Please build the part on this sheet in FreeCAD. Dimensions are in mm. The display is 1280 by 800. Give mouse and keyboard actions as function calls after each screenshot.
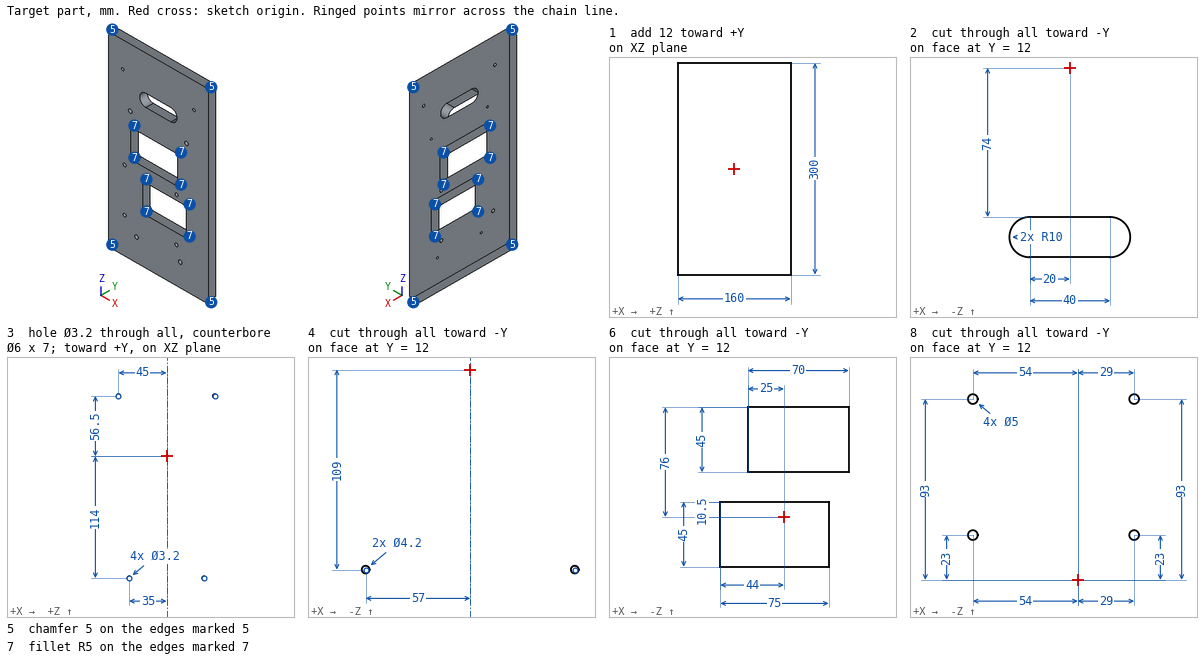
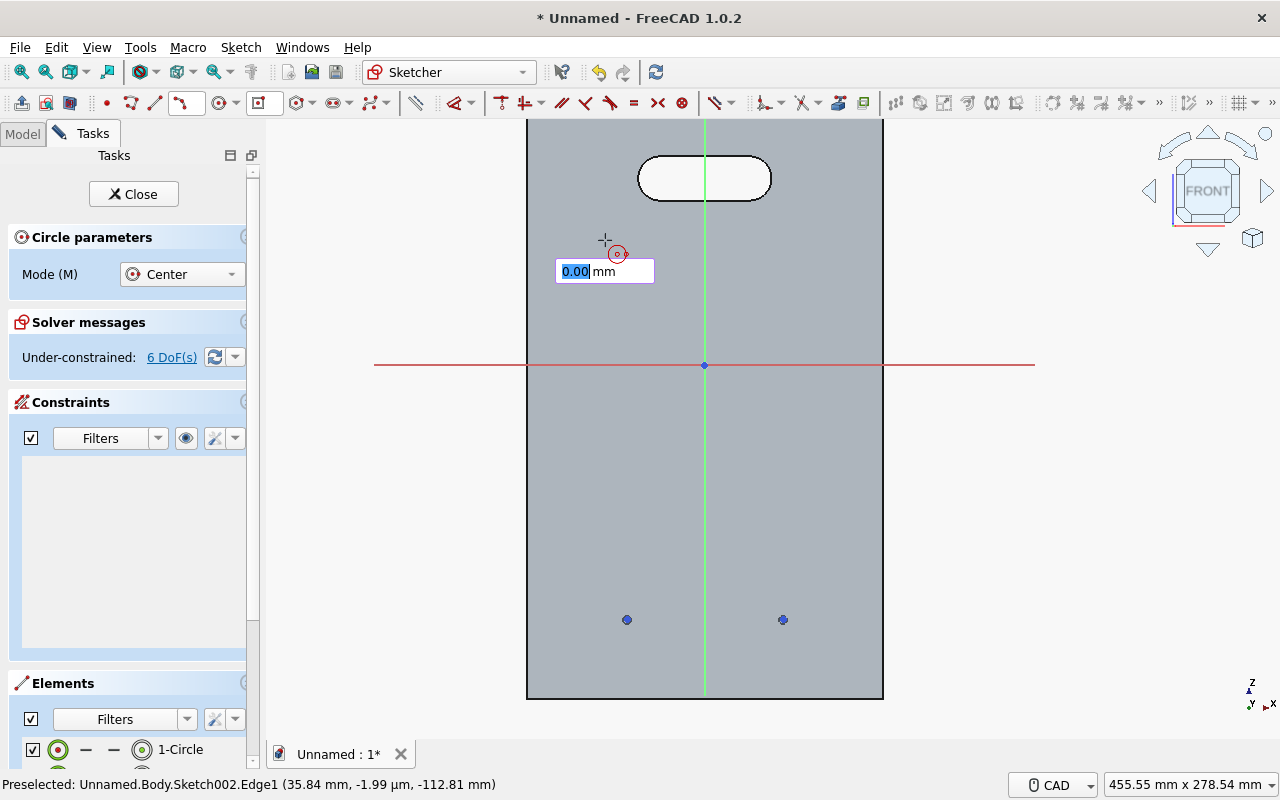
scroll(607, 237, up, 8)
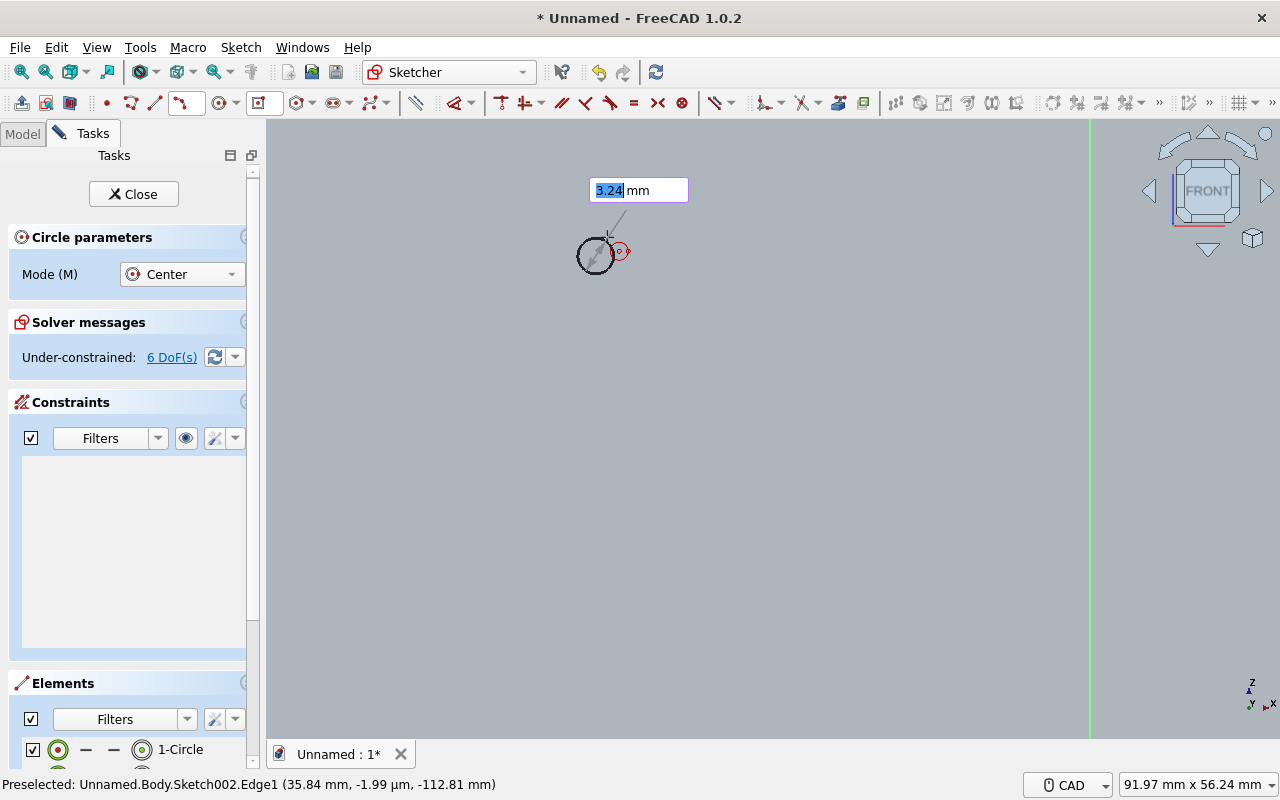
click(607, 237)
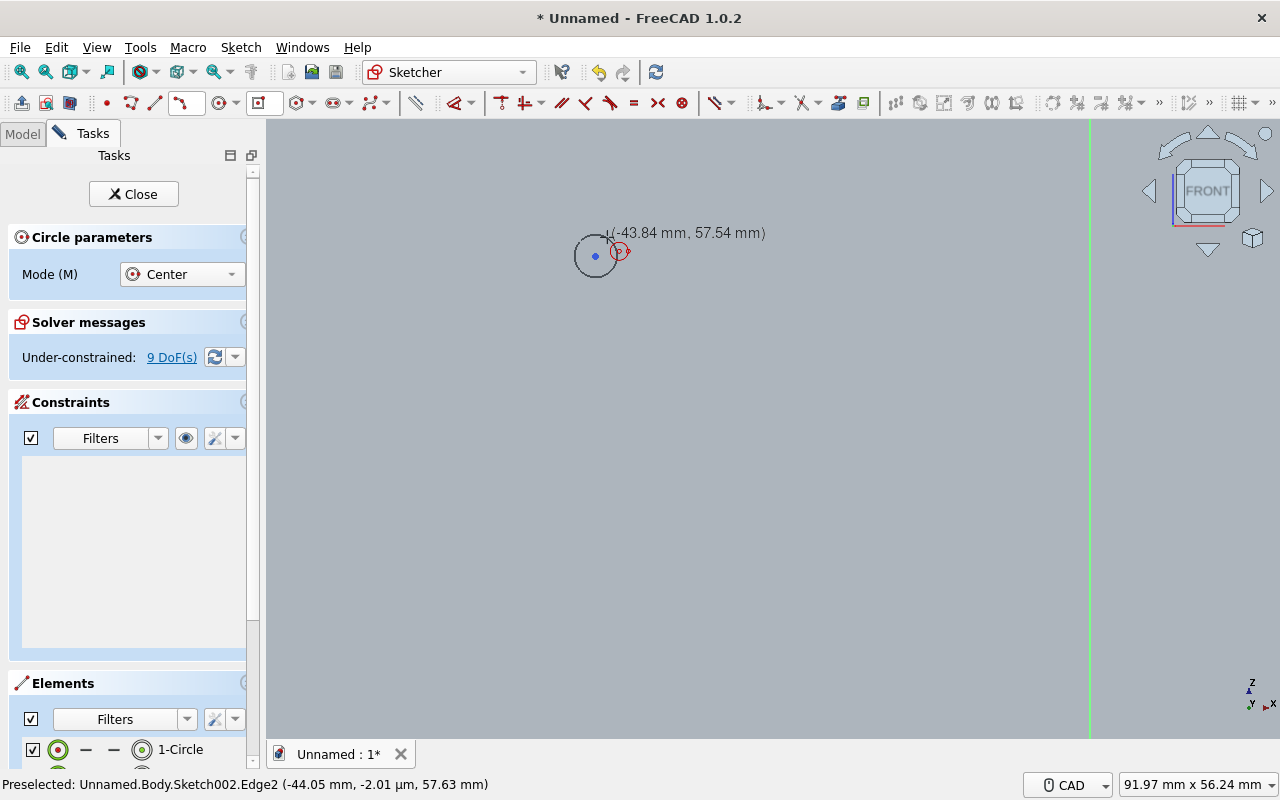
scroll(607, 237, down, 8)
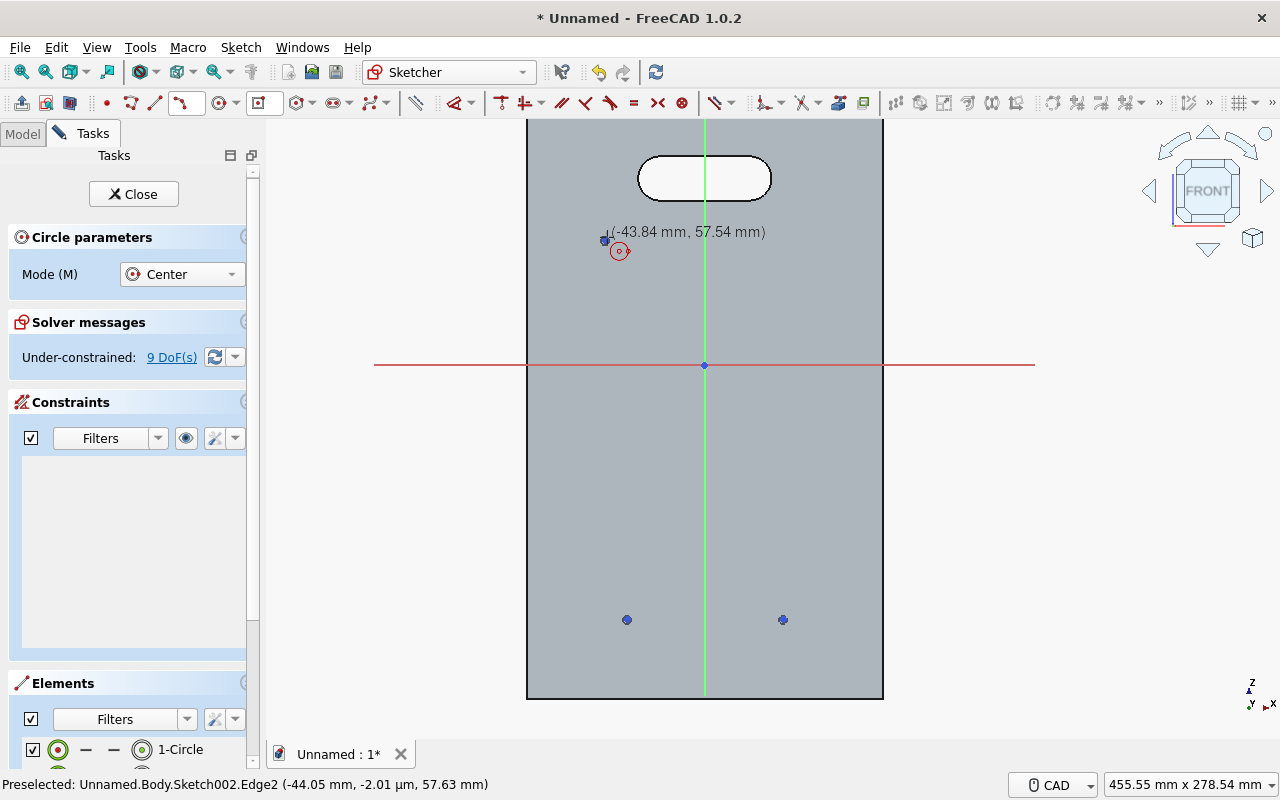
scroll(805, 240, up, 10)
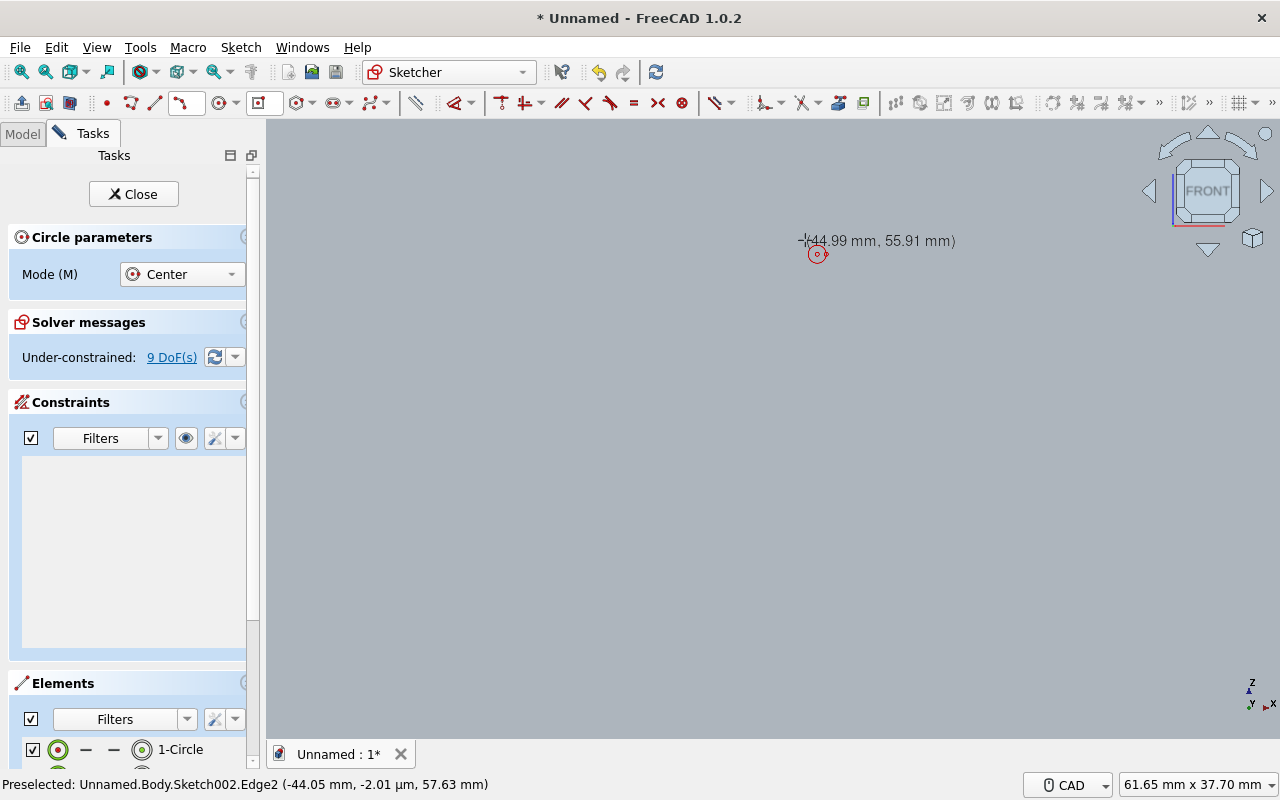
scroll(805, 240, down, 10)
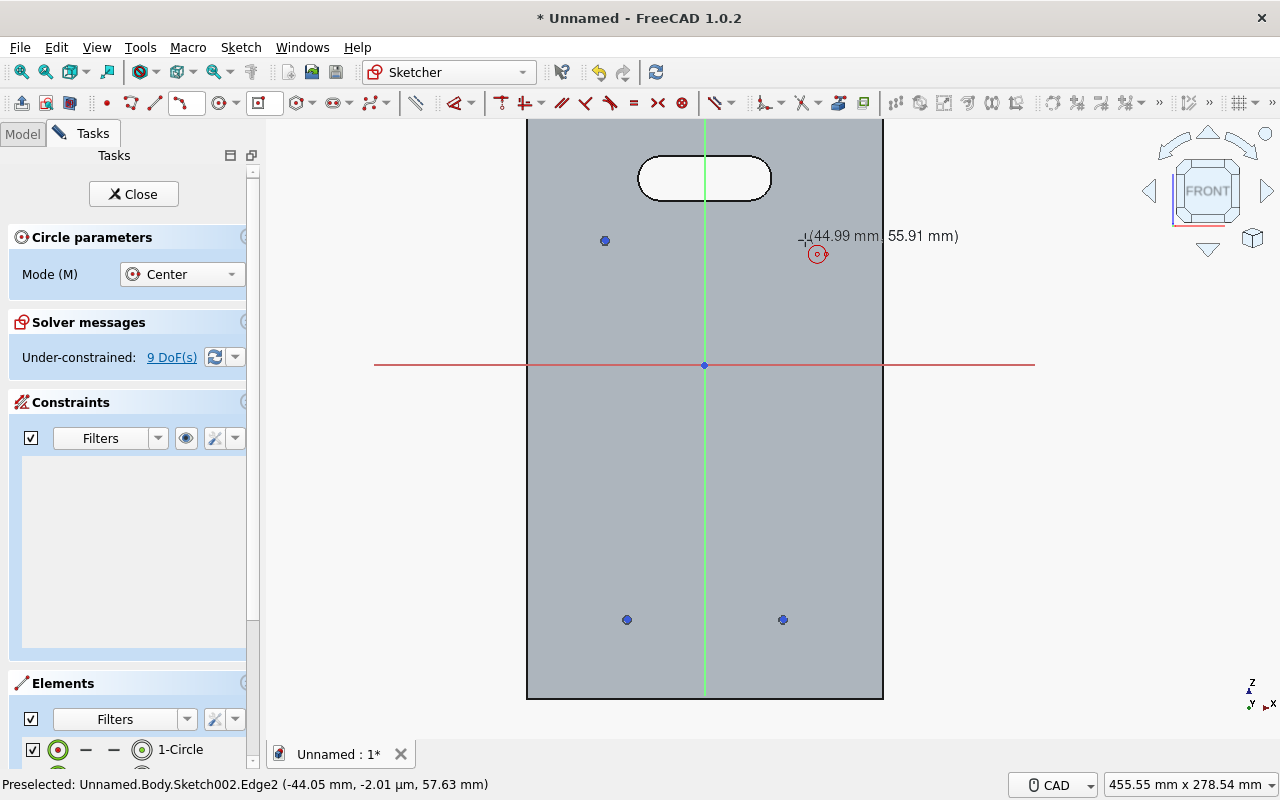
click(805, 240)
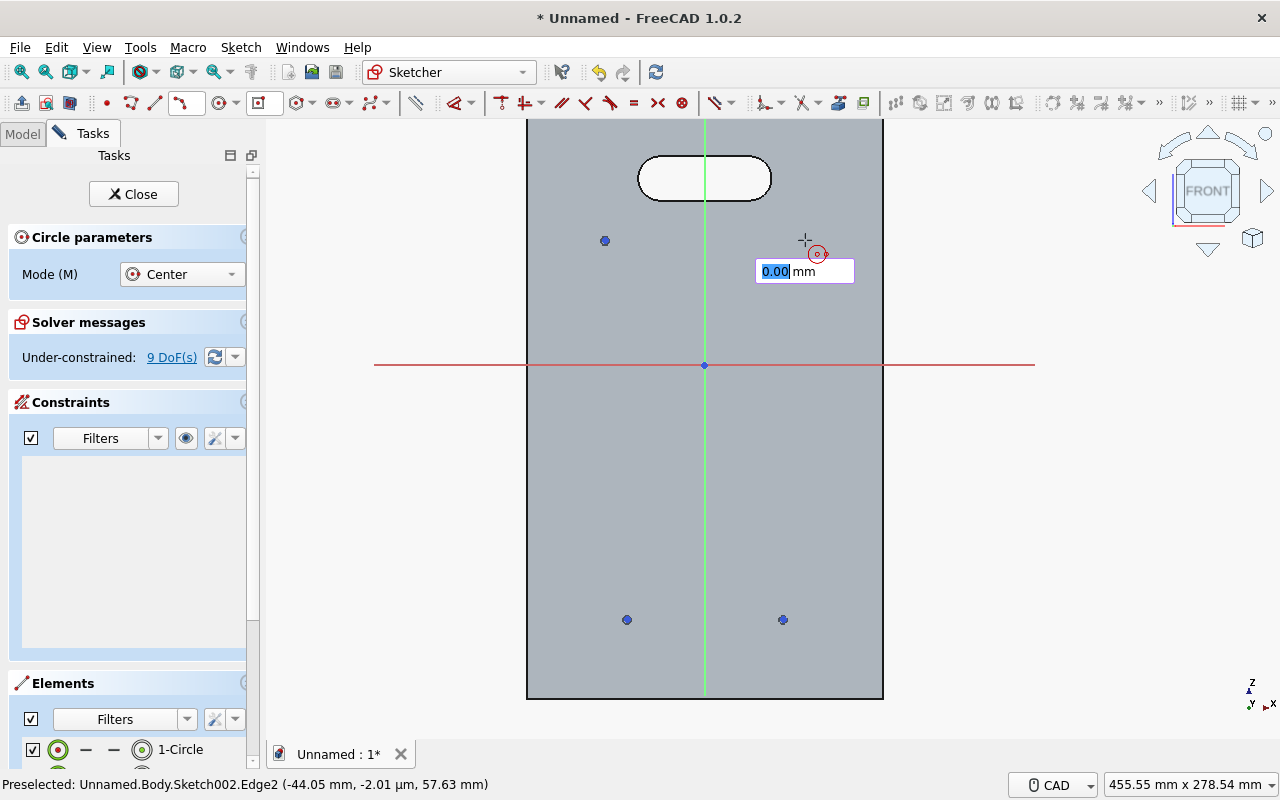
scroll(808, 237, up, 8)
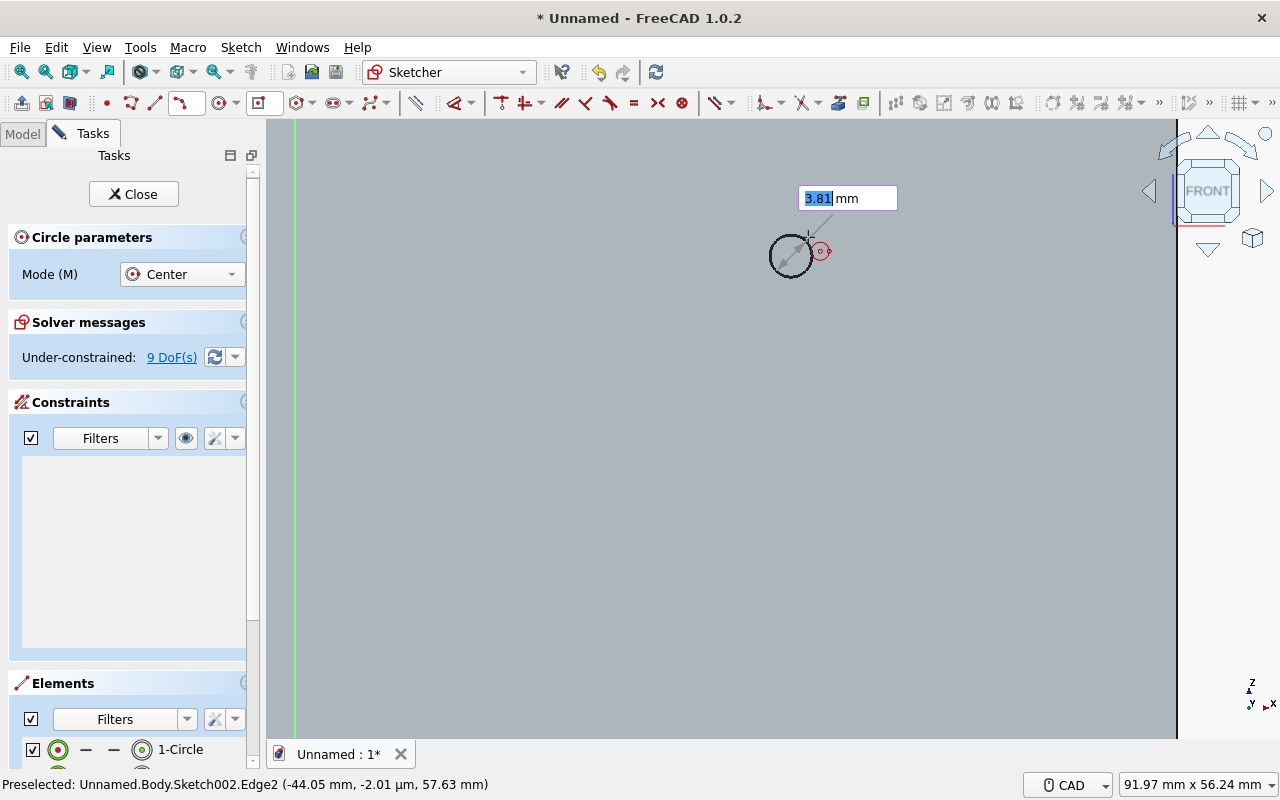
click(804, 237)
key(Escape)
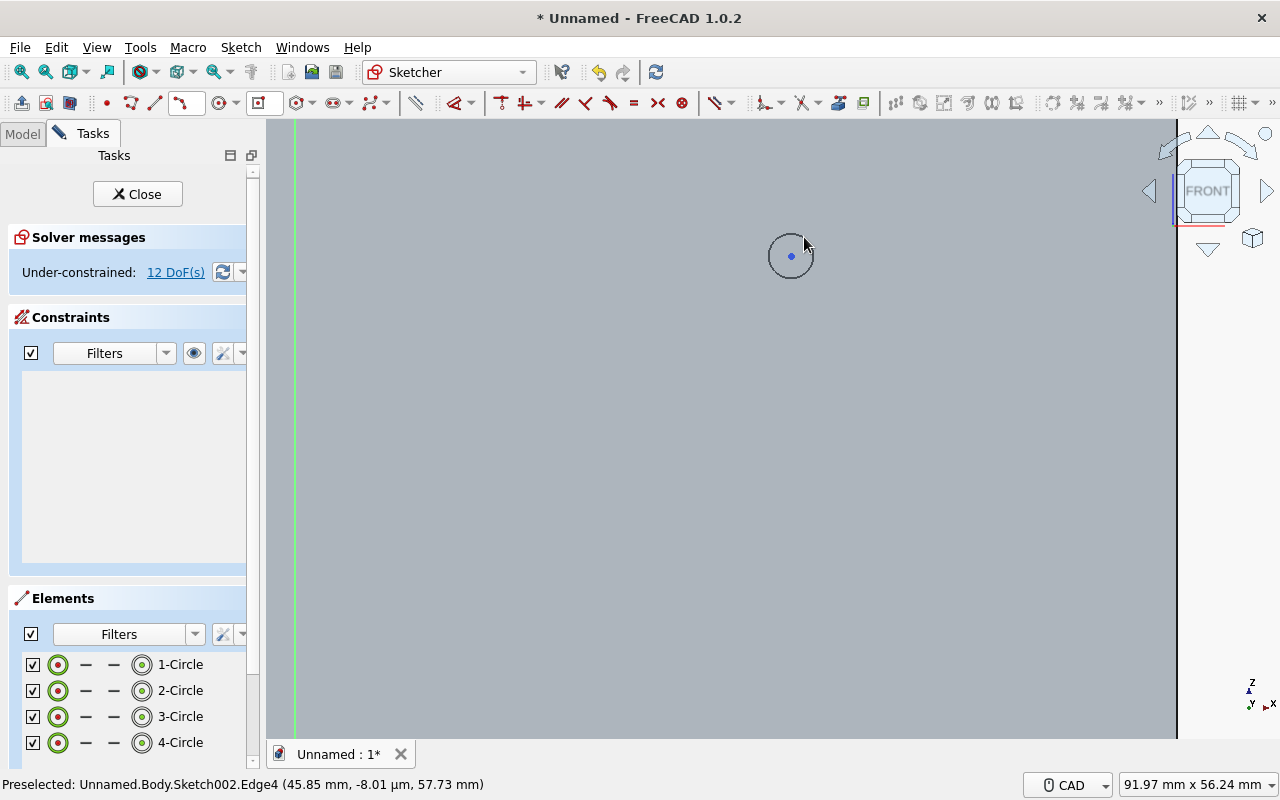
scroll(808, 237, down, 8)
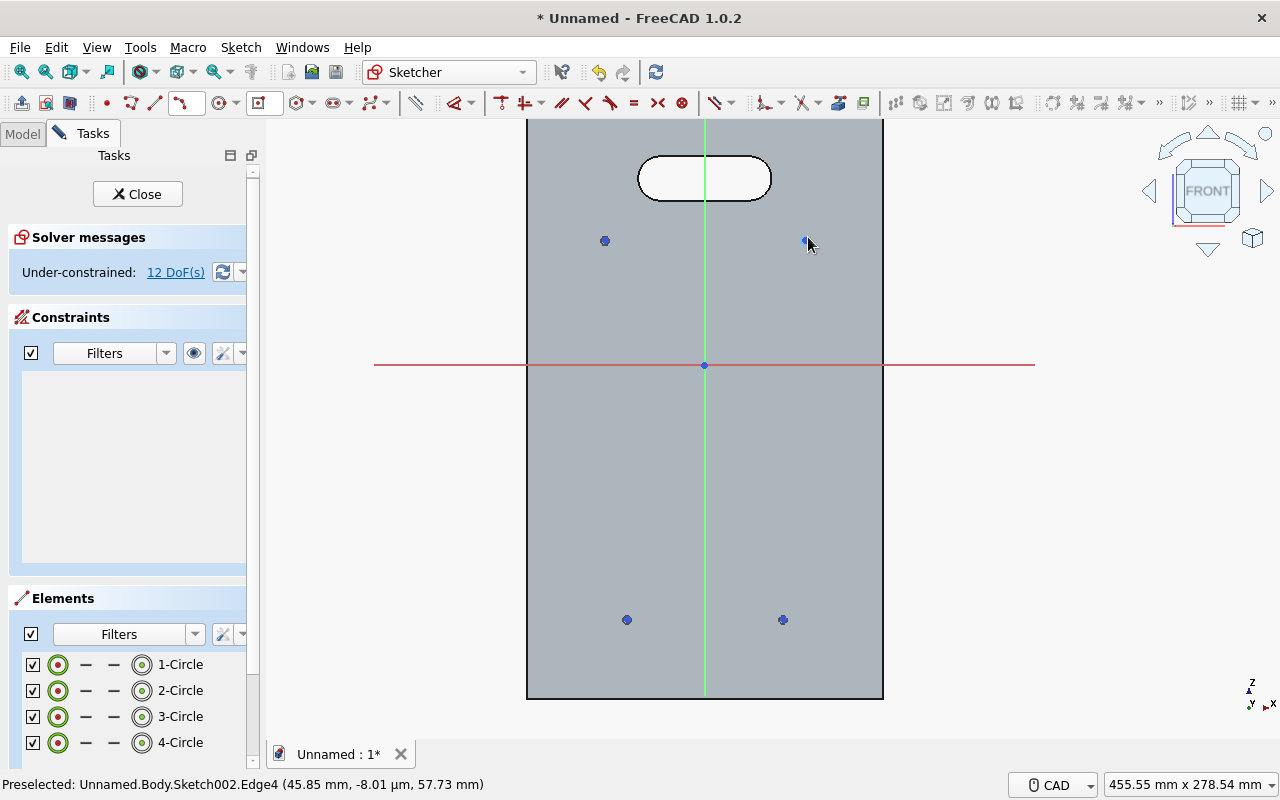
scroll(630, 617, up, 7)